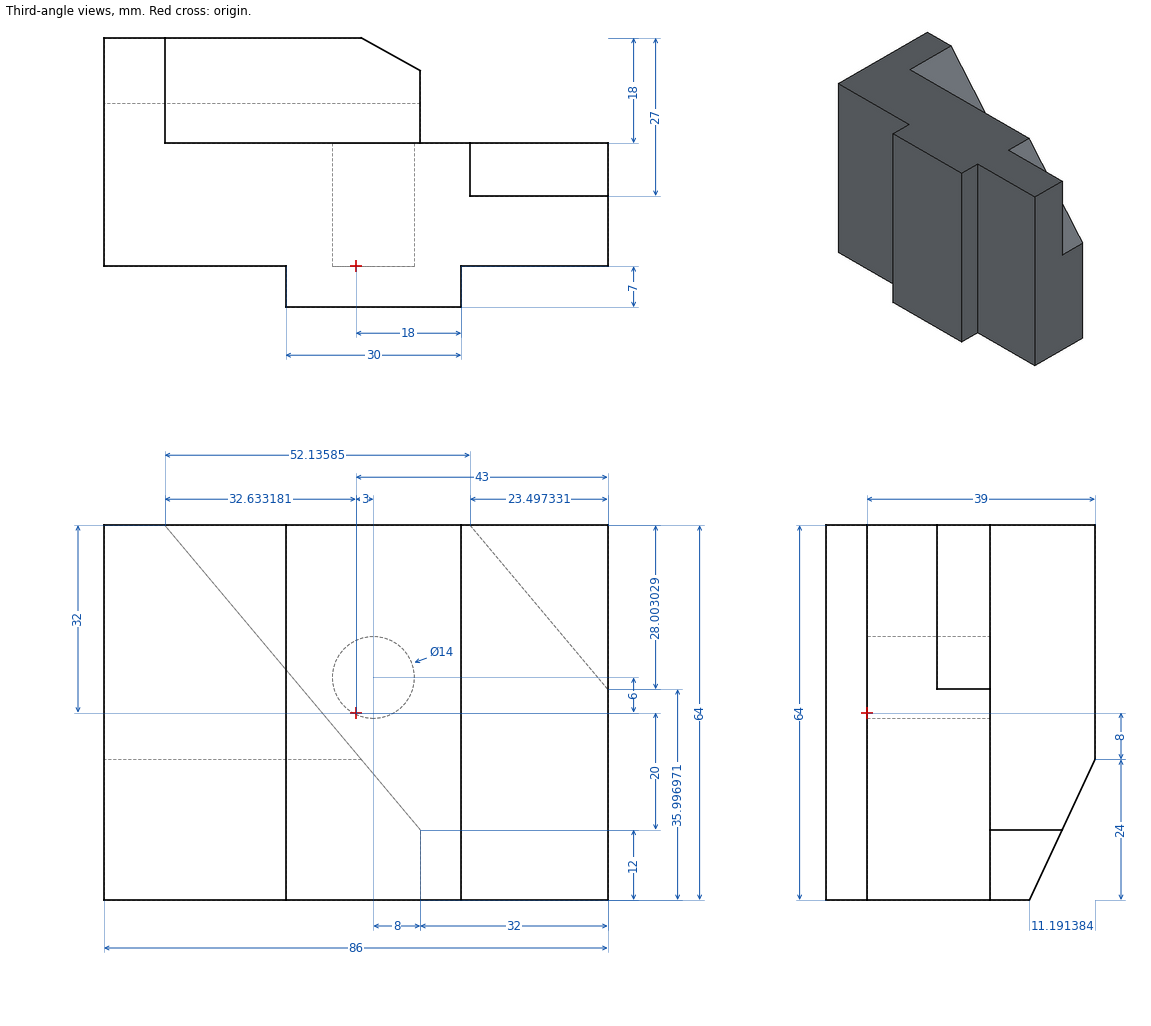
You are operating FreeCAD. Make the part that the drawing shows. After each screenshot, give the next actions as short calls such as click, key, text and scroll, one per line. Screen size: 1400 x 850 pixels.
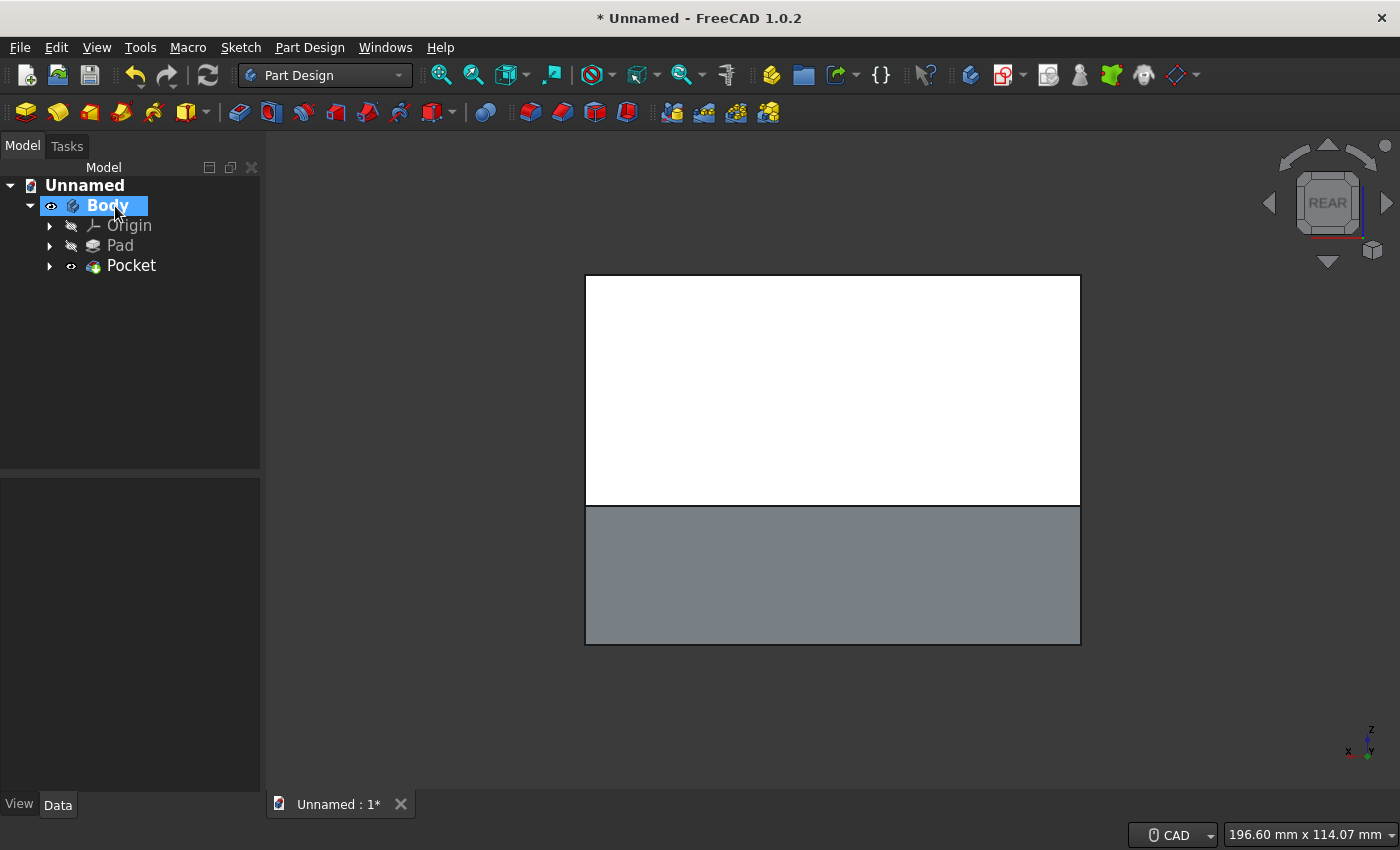
click(762, 390)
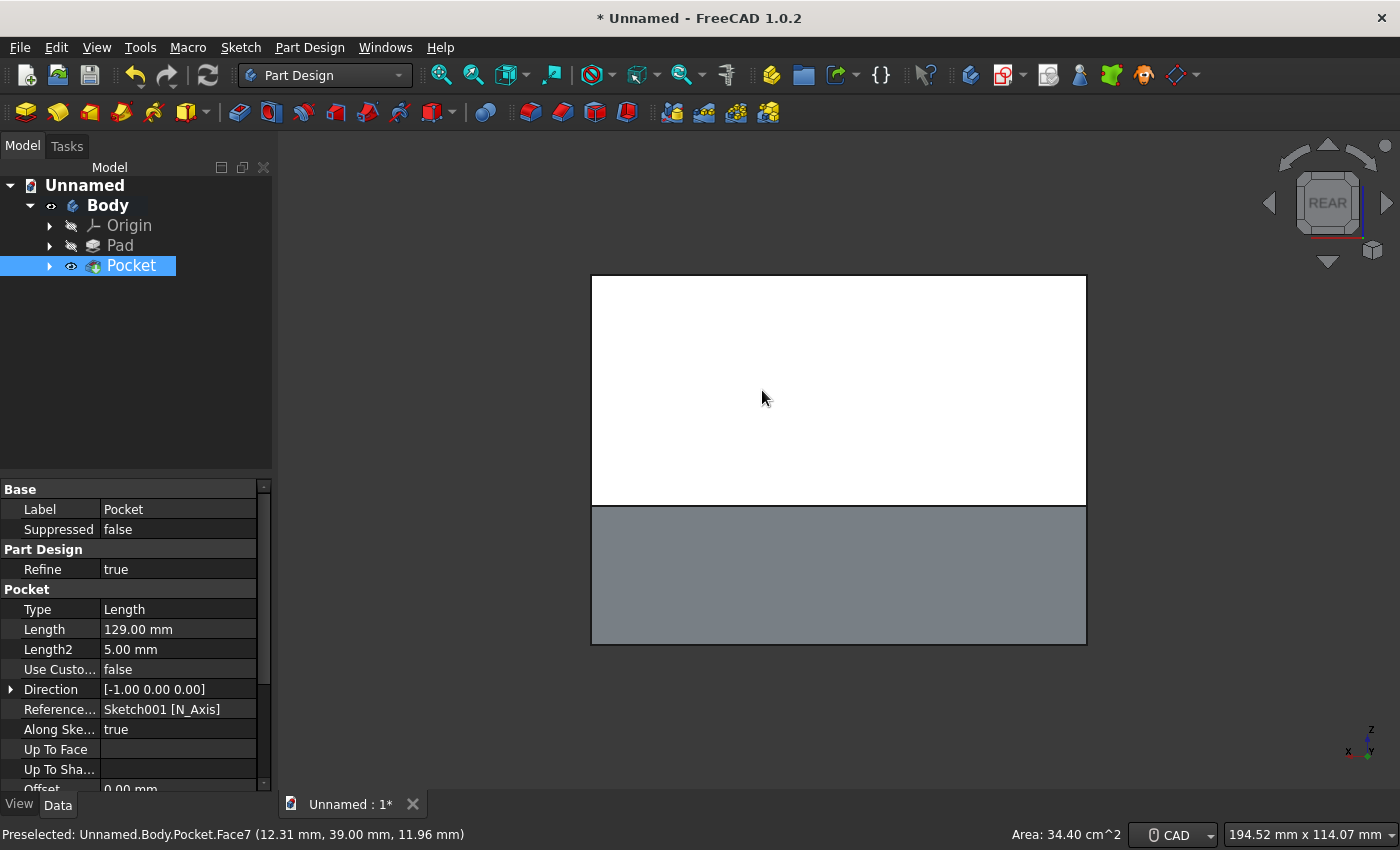
click(1004, 76)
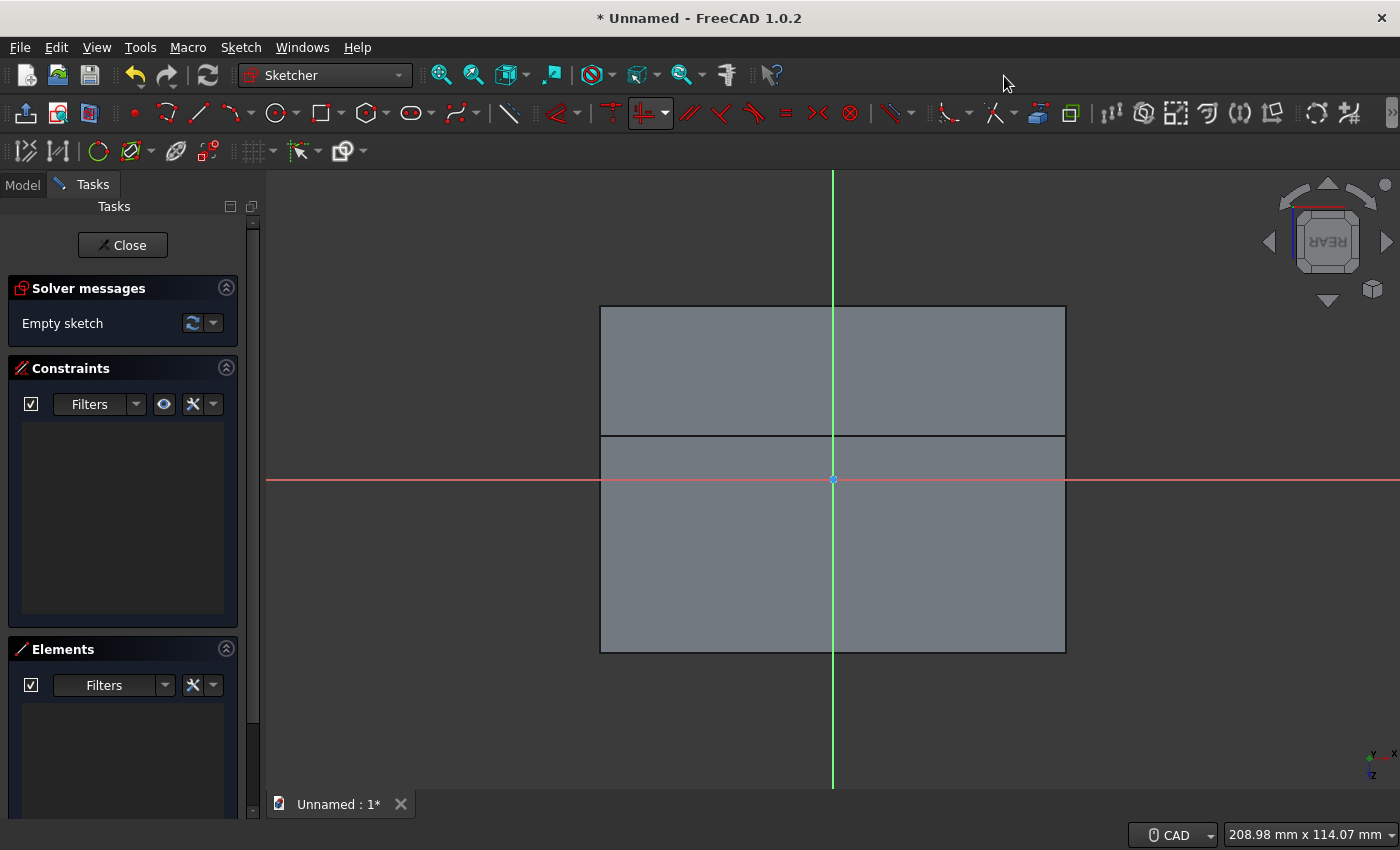
key(g)
key(m)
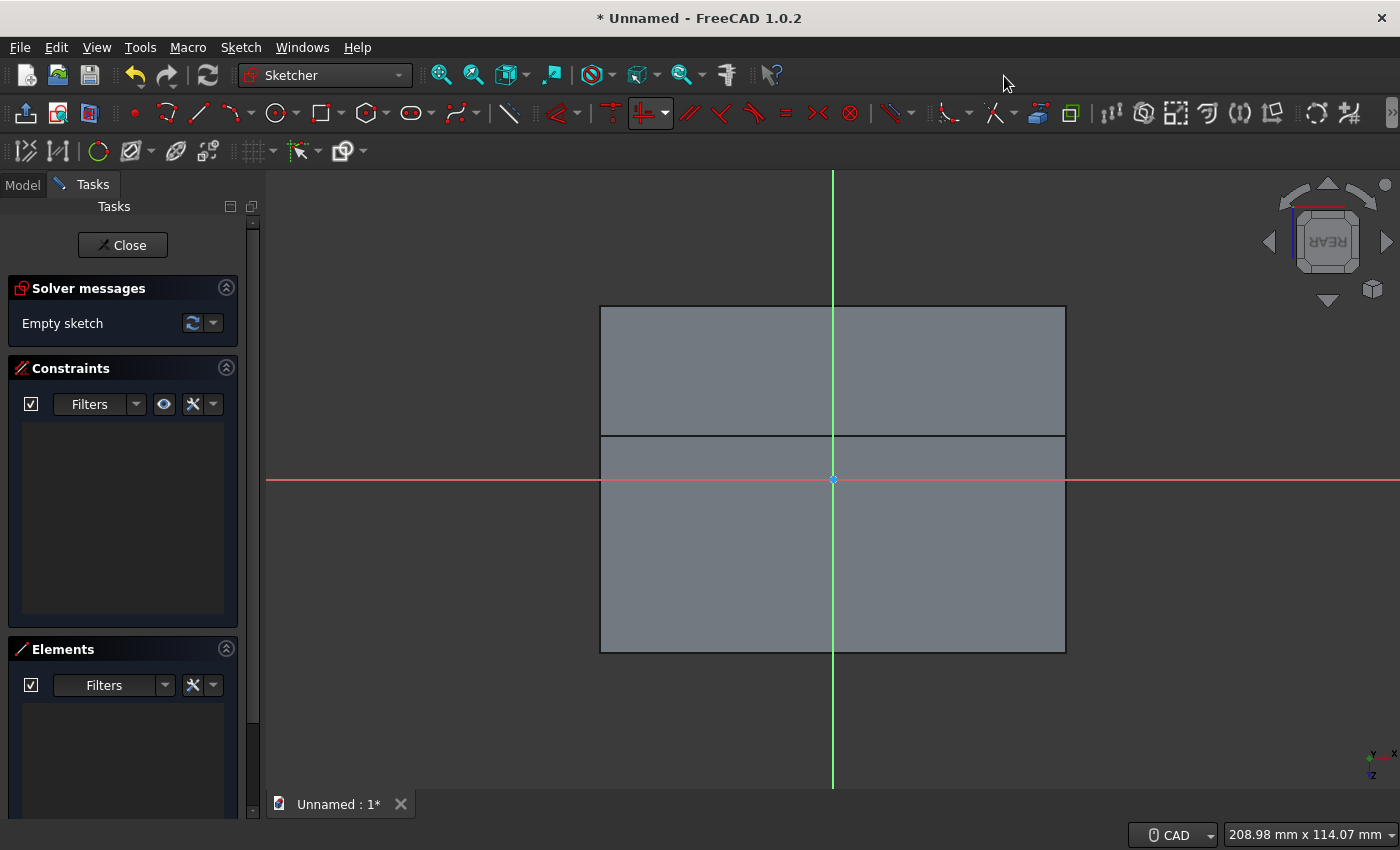
click(893, 371)
click(656, 653)
click(939, 653)
click(1066, 501)
click(1066, 306)
click(893, 306)
click(893, 372)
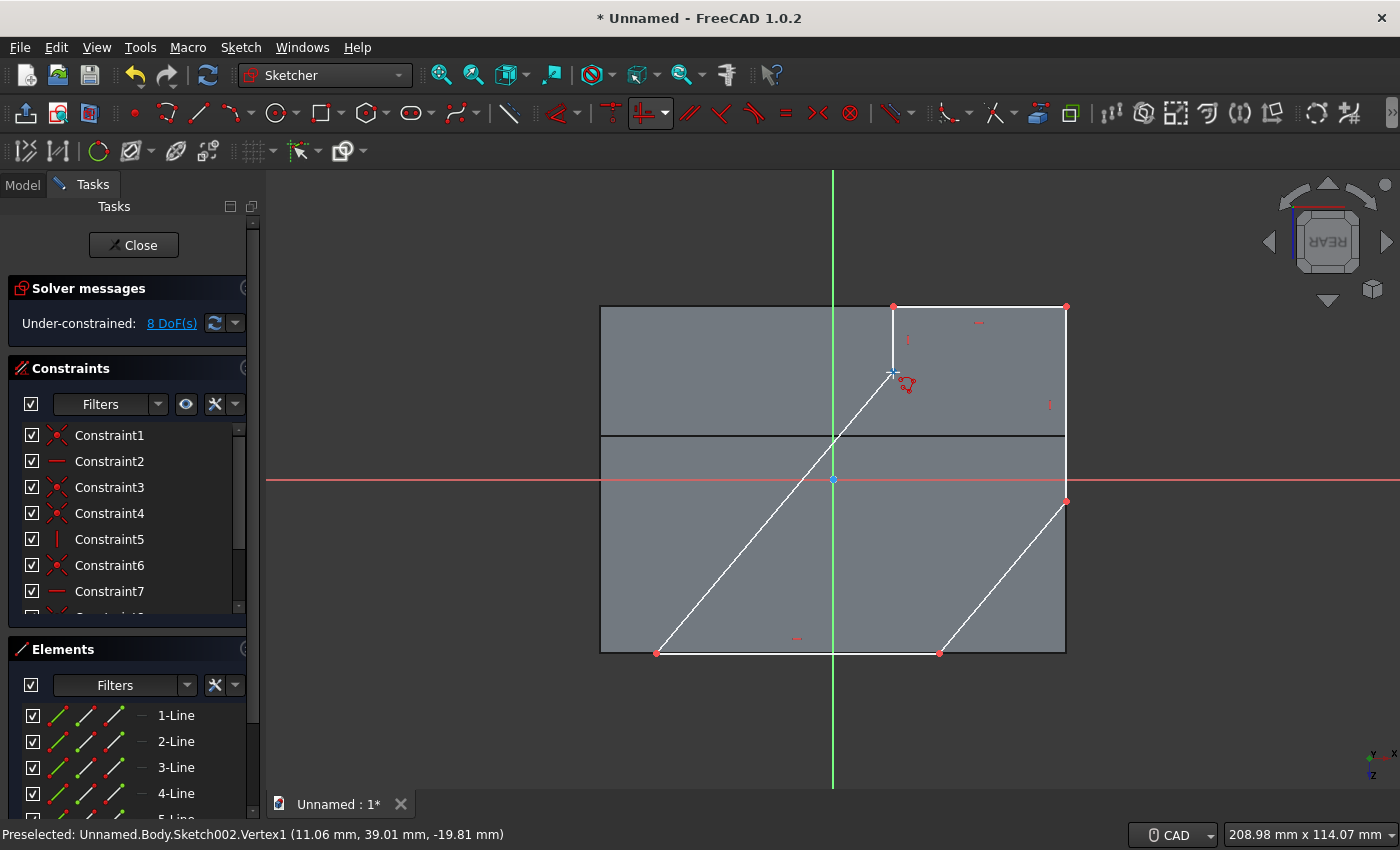
click(276, 114)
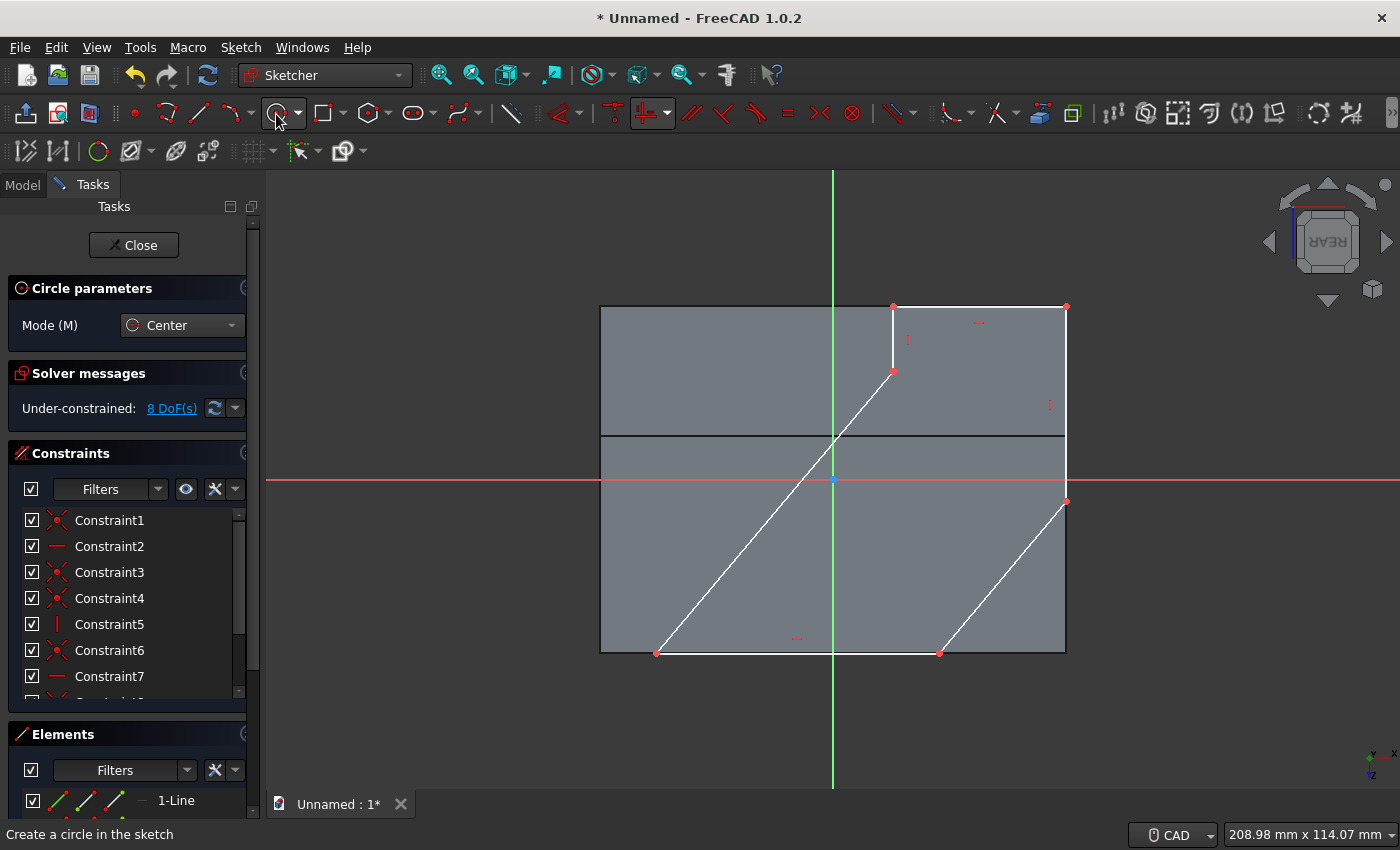
click(849, 512)
move(876, 539)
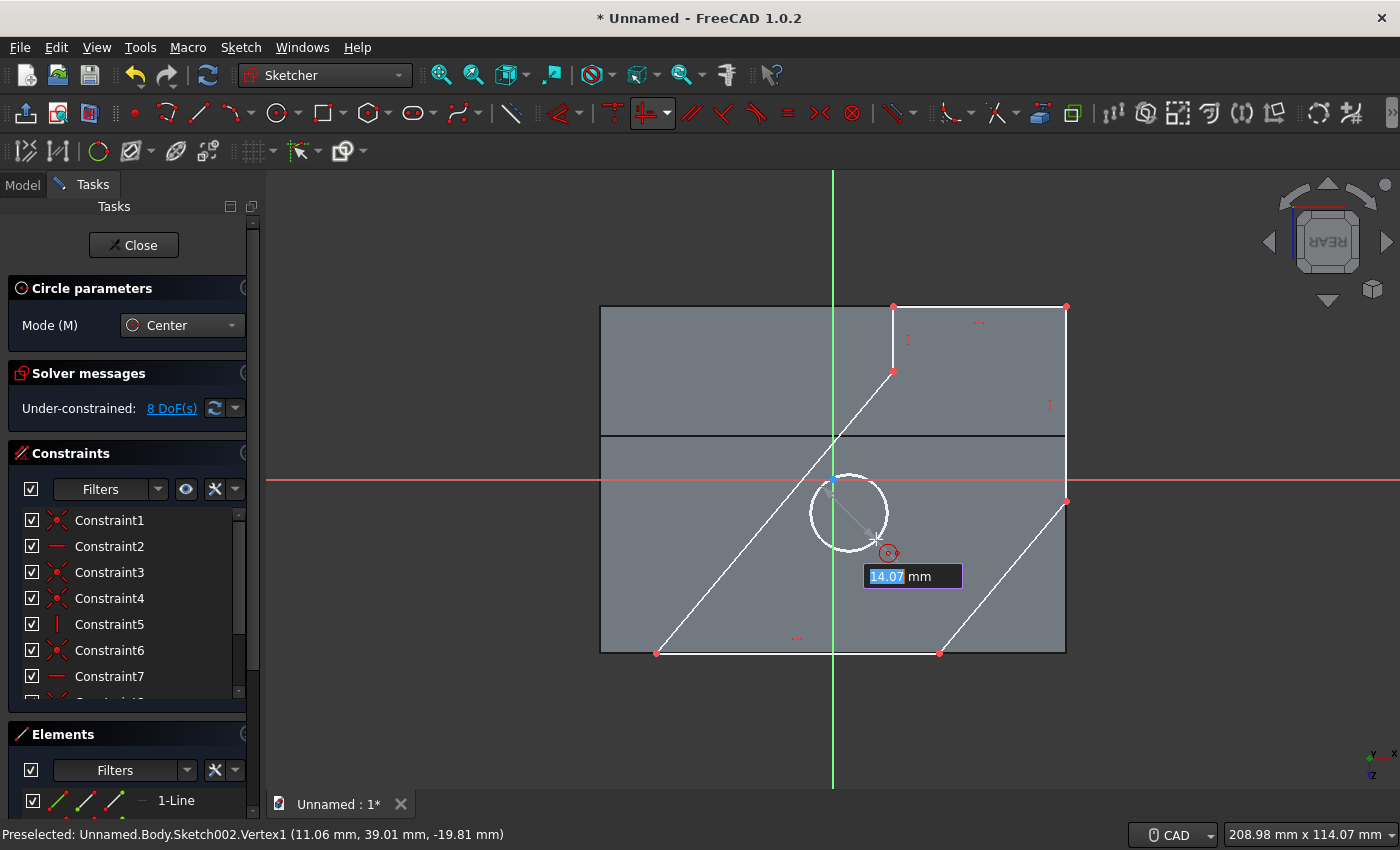
text(14)
key(Return)
key(Escape)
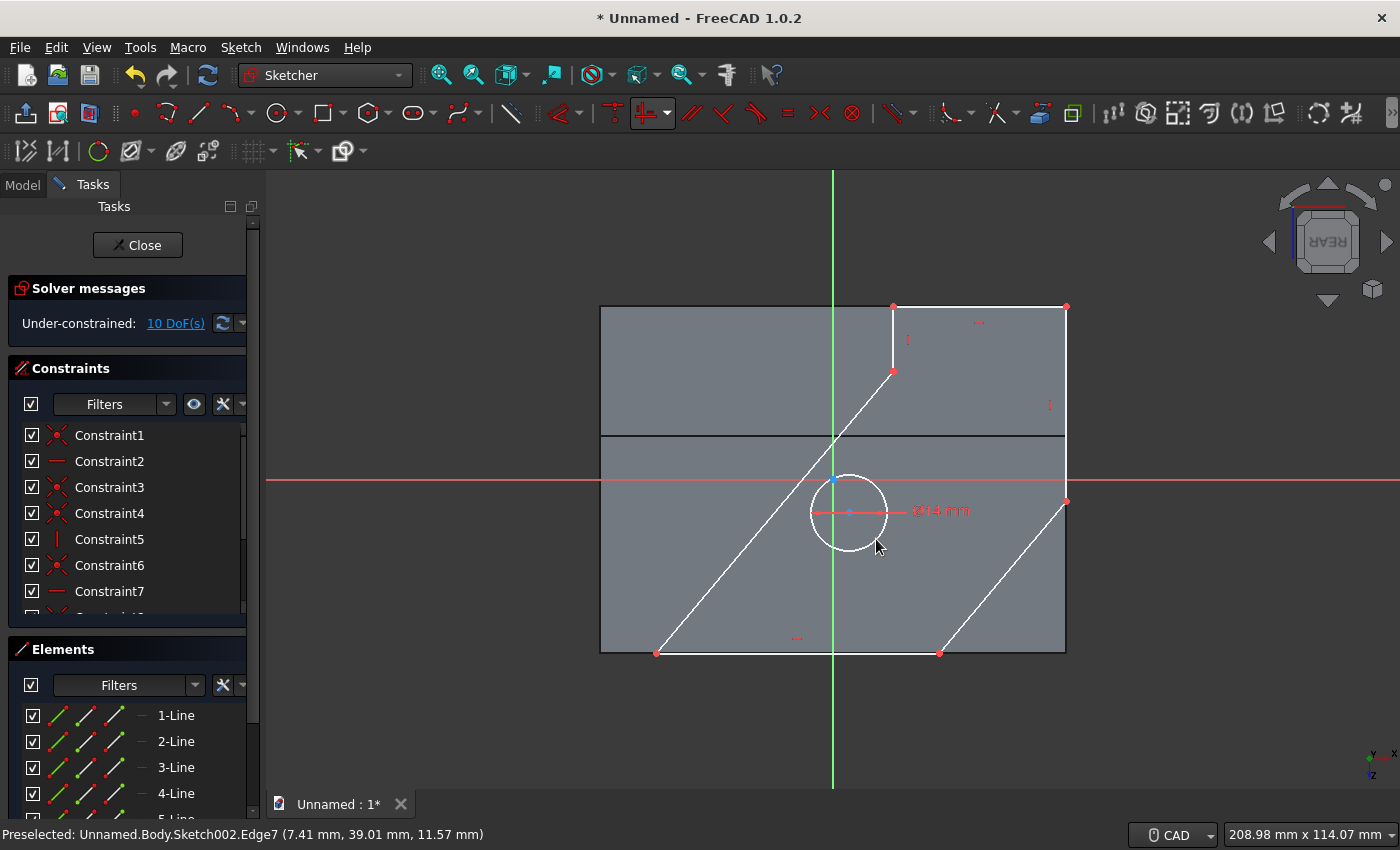
click(558, 114)